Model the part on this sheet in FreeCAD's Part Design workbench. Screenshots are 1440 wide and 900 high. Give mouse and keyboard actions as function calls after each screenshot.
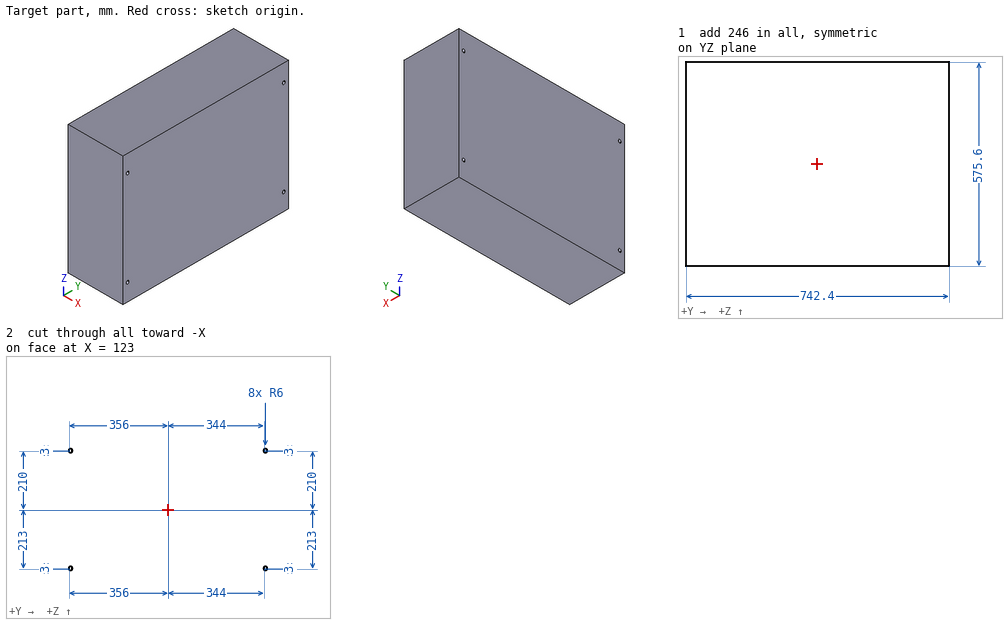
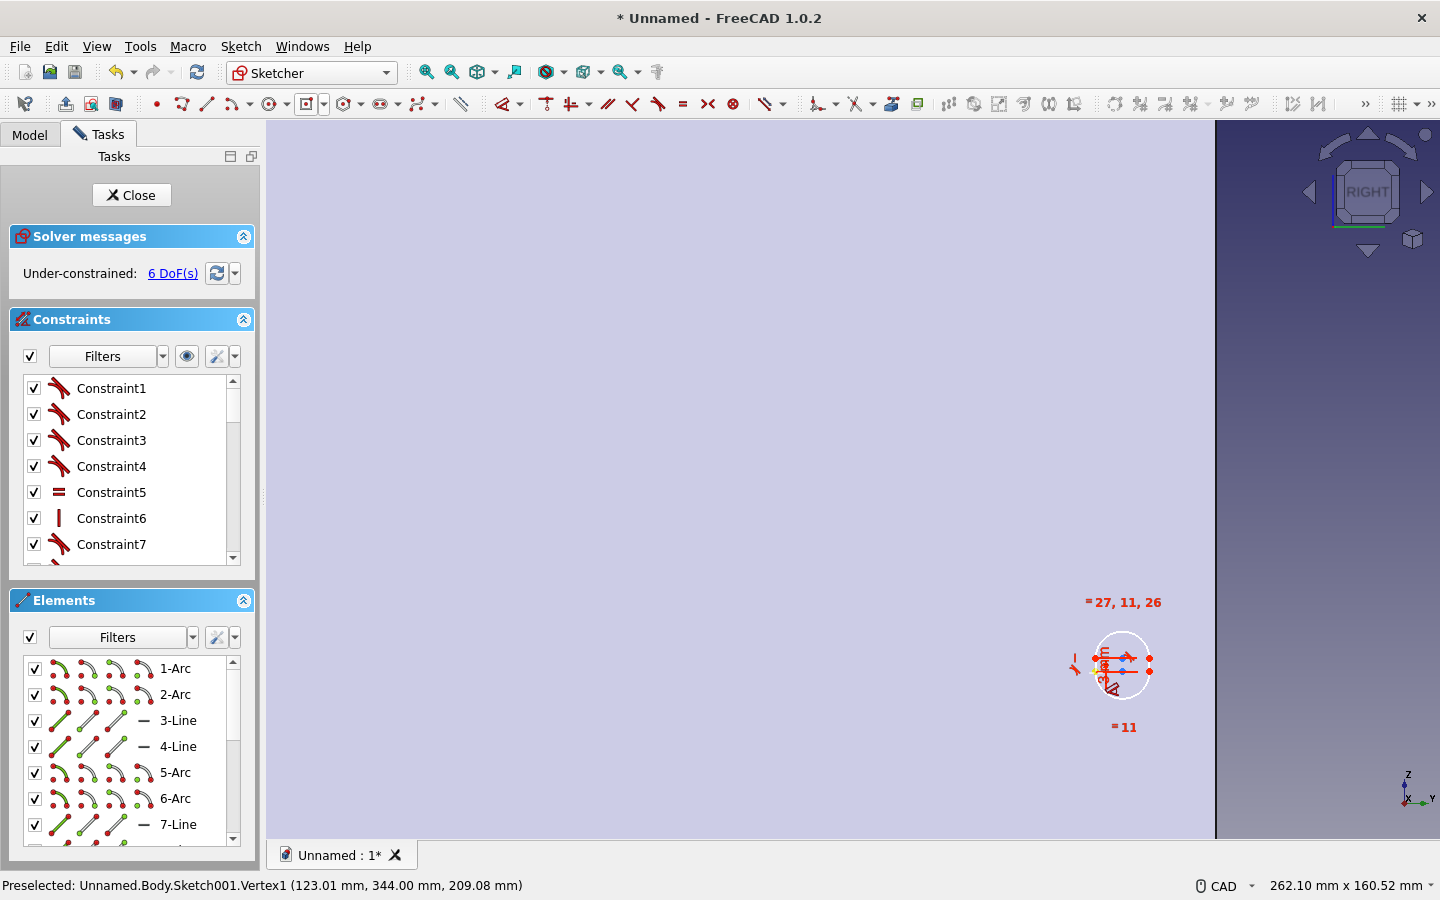
click(1096, 672)
click(695, 706)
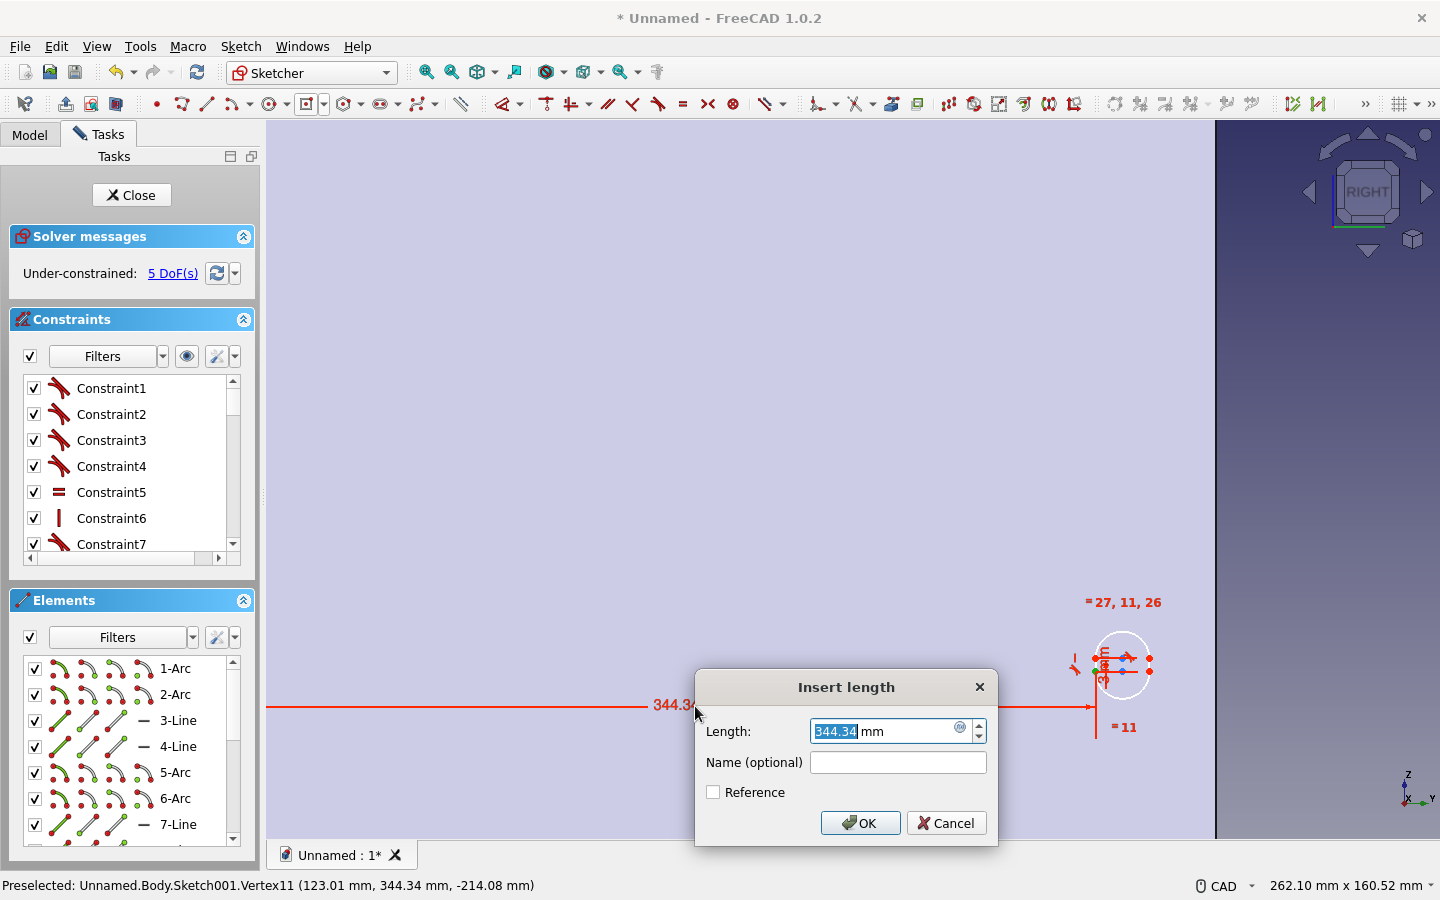
text(344)
key(Return)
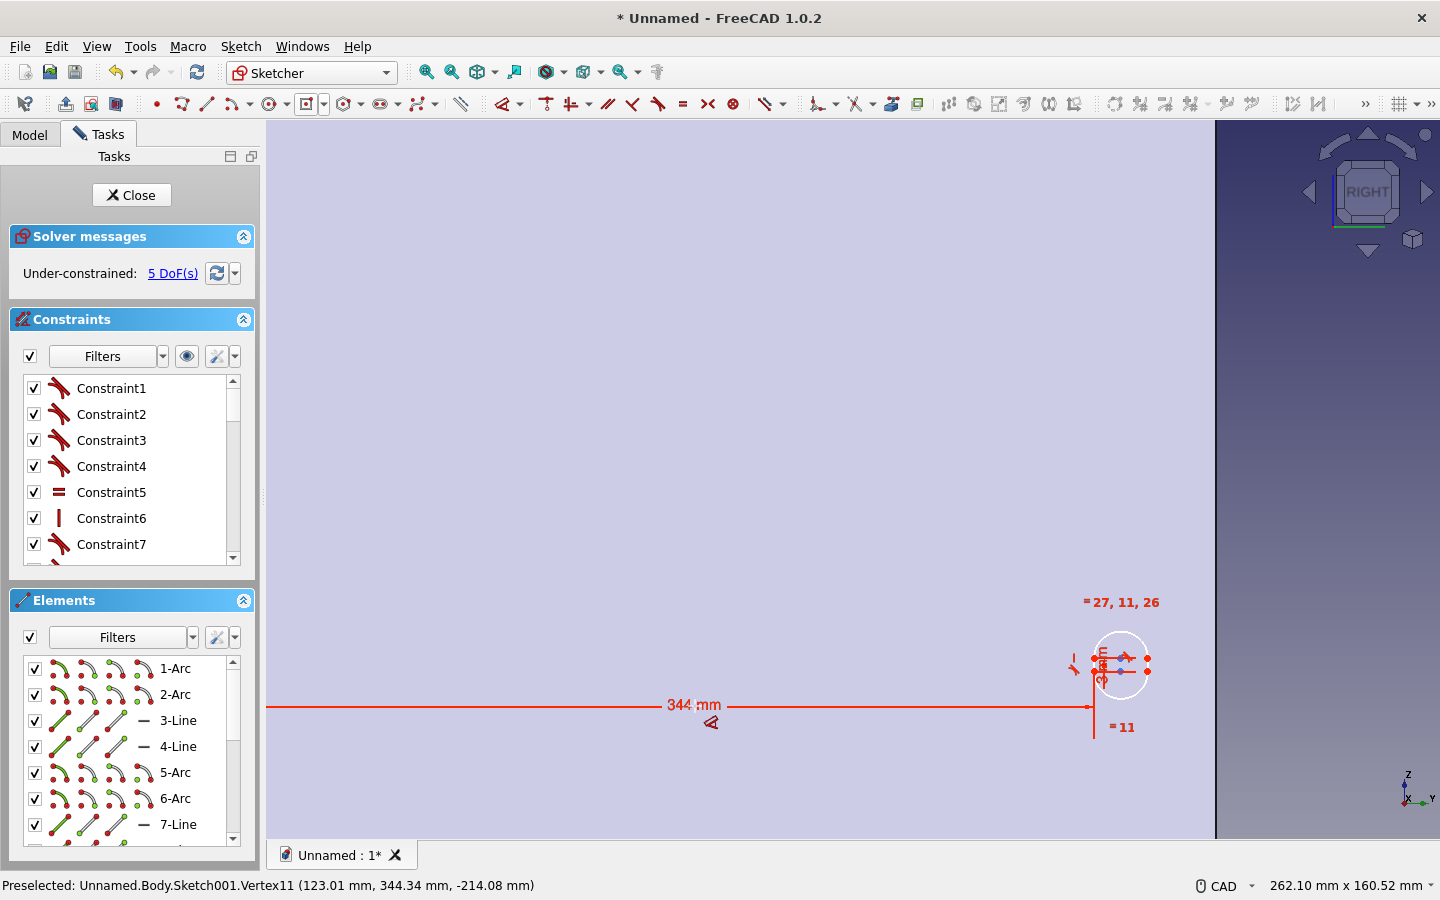
click(1094, 672)
click(1128, 410)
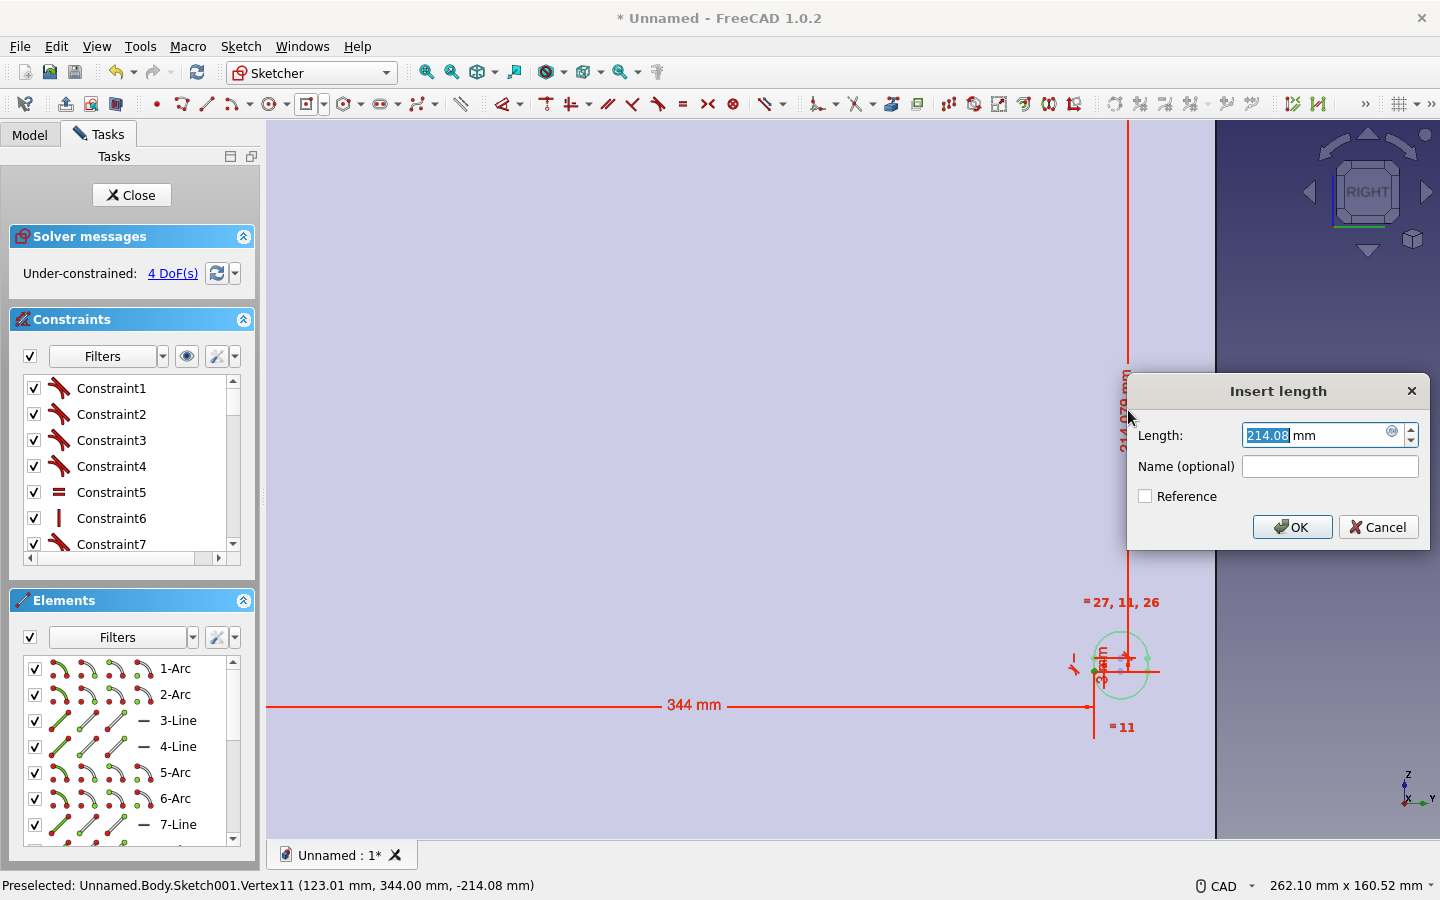
text(213)
key(Return)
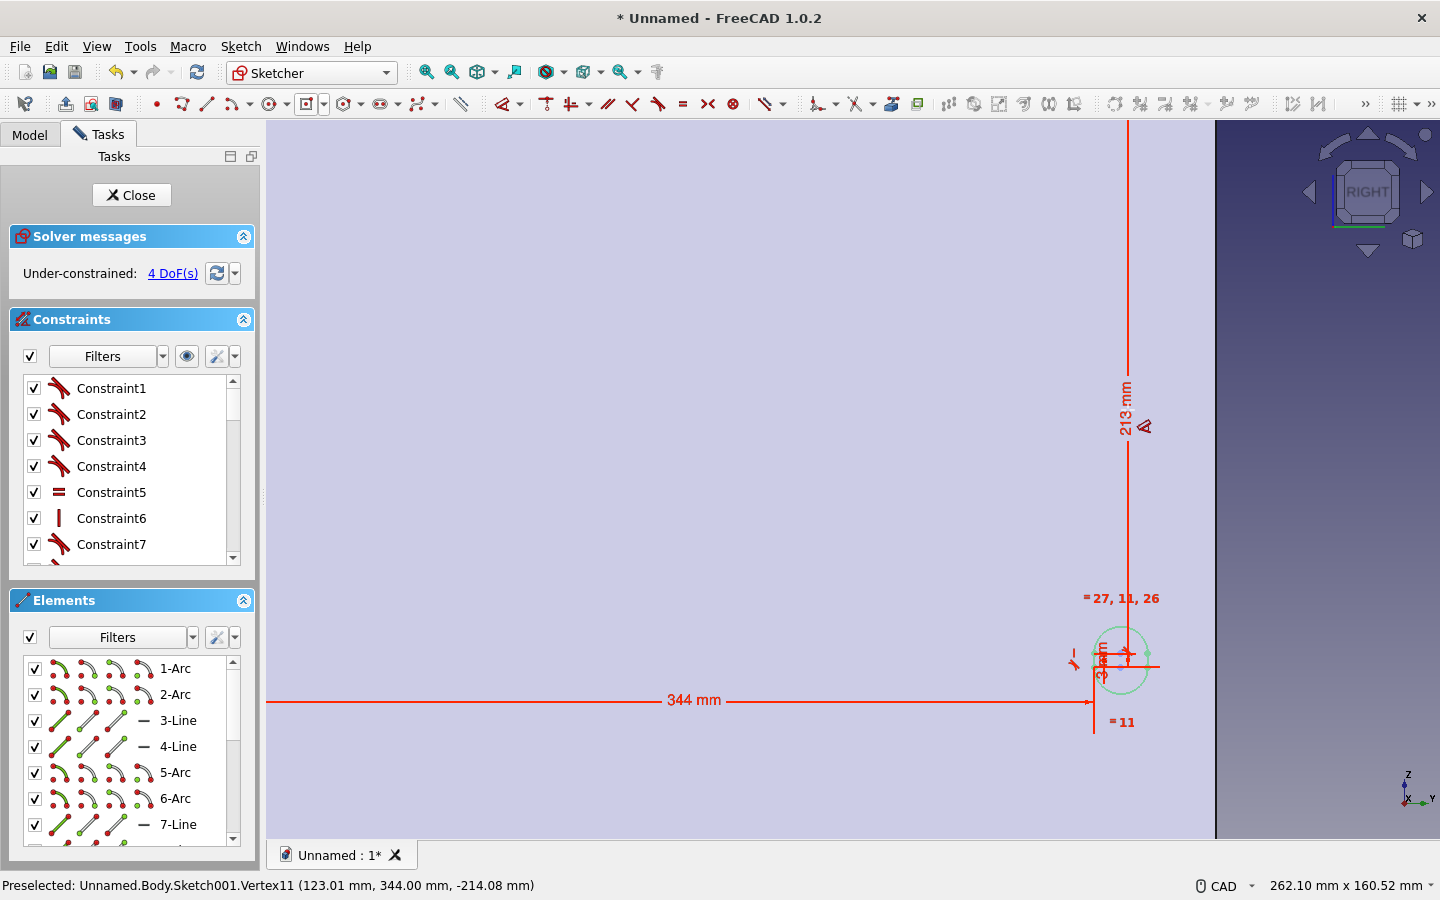
scroll(1096, 673, down, 8)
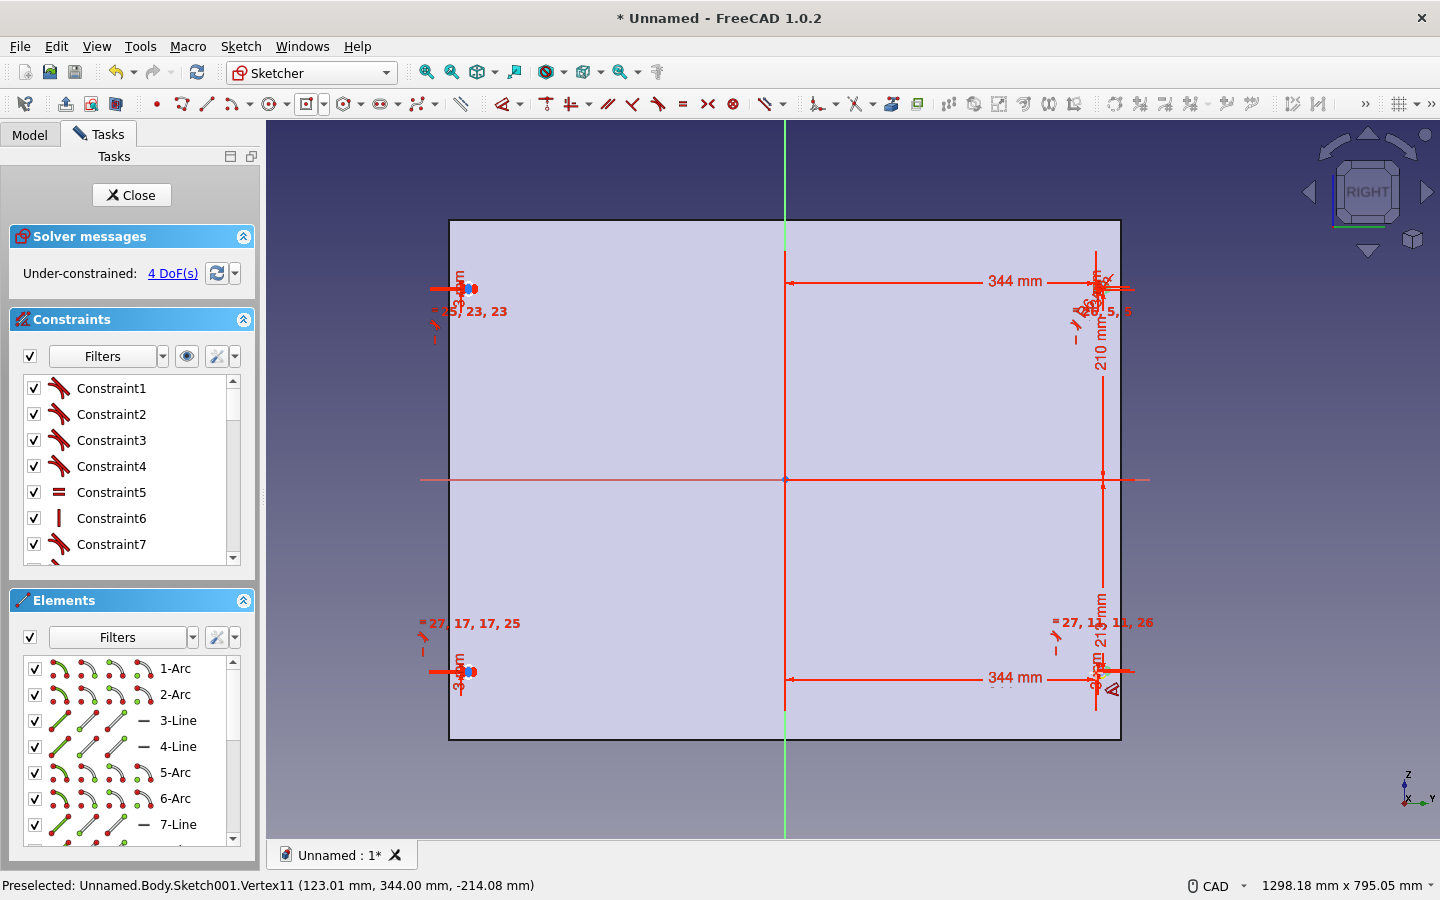
scroll(463, 673, up, 8)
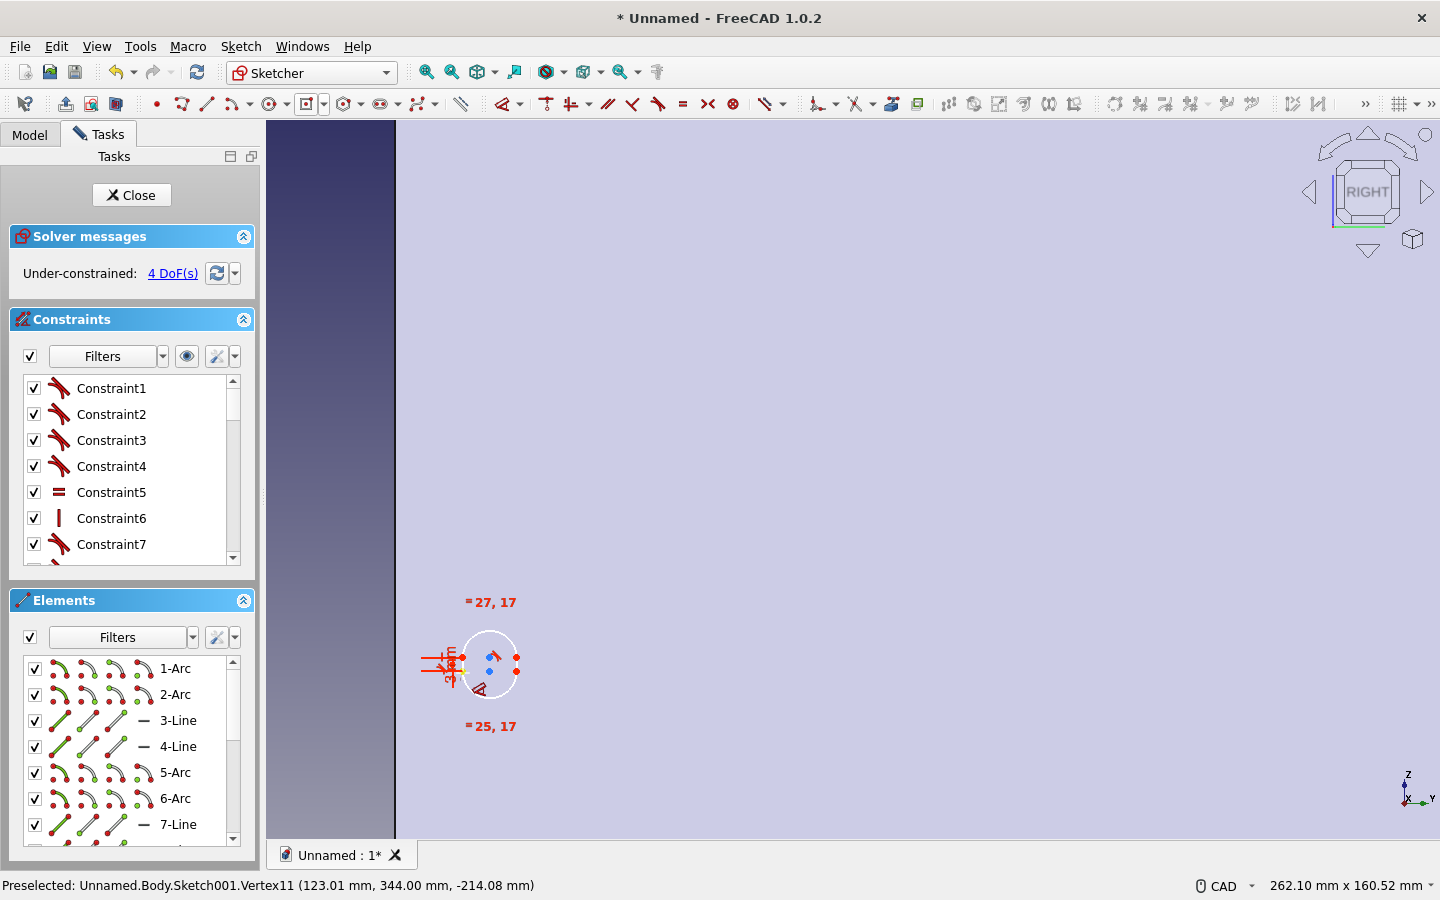
click(463, 671)
click(869, 705)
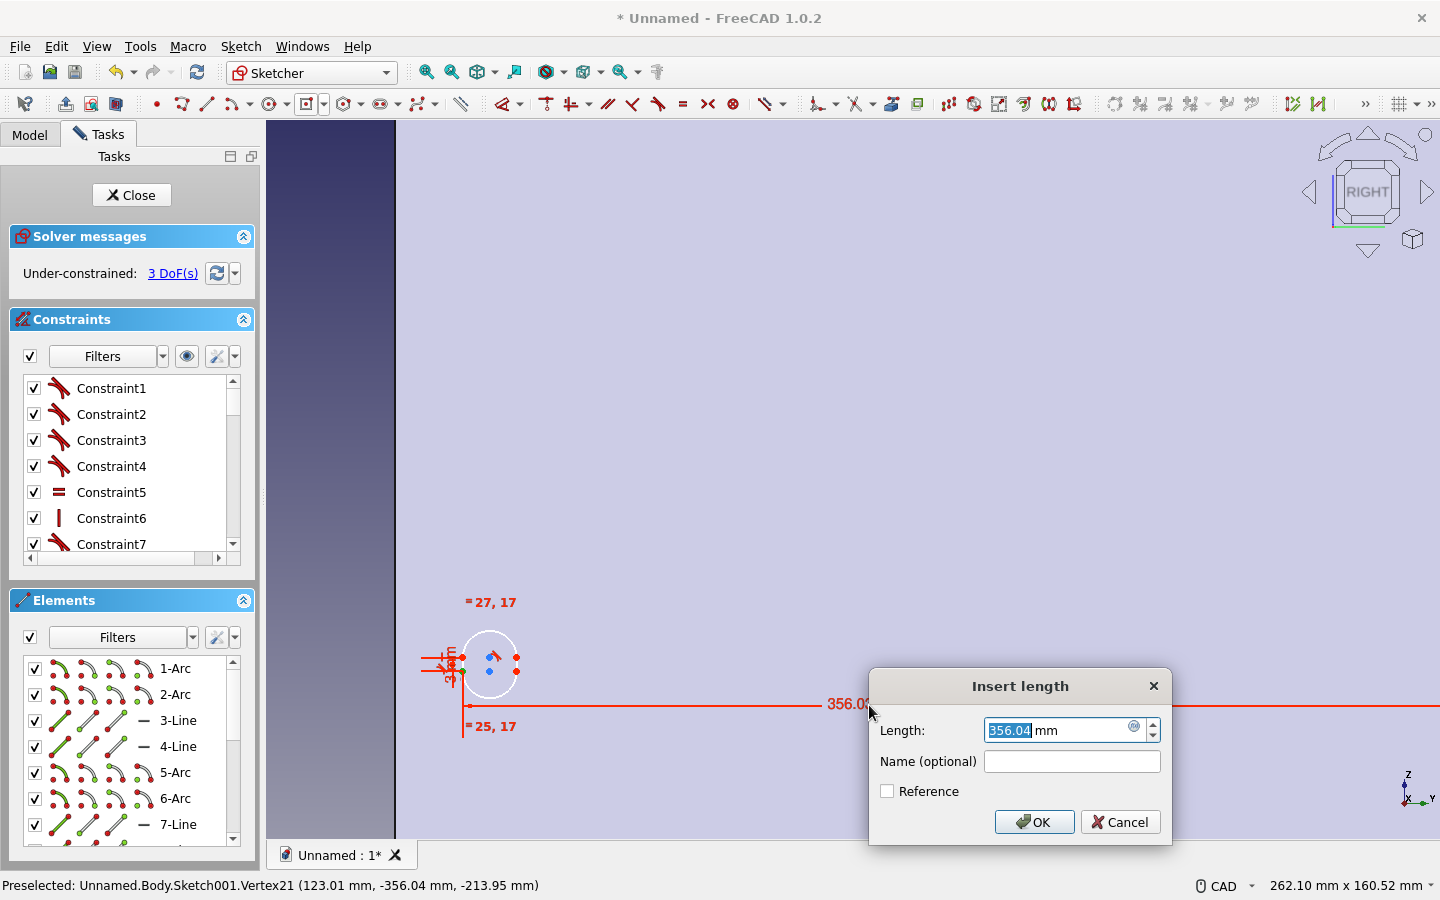
text(356)
key(Return)